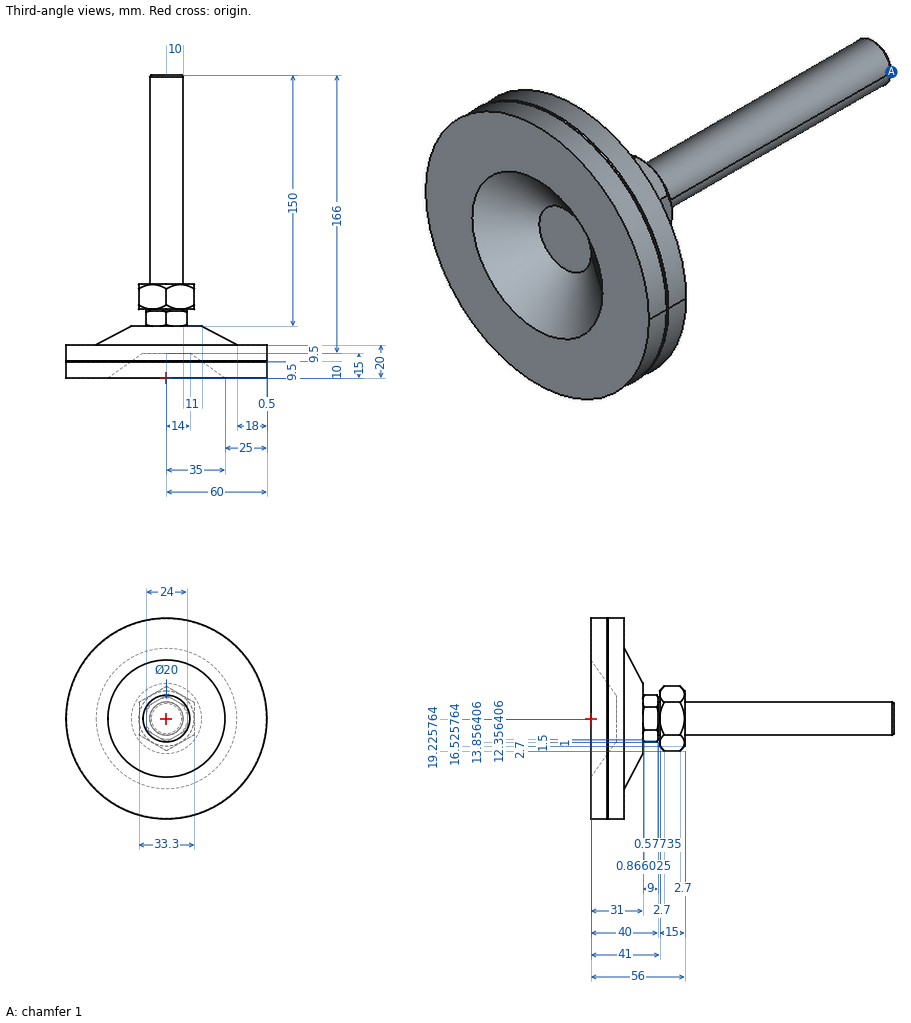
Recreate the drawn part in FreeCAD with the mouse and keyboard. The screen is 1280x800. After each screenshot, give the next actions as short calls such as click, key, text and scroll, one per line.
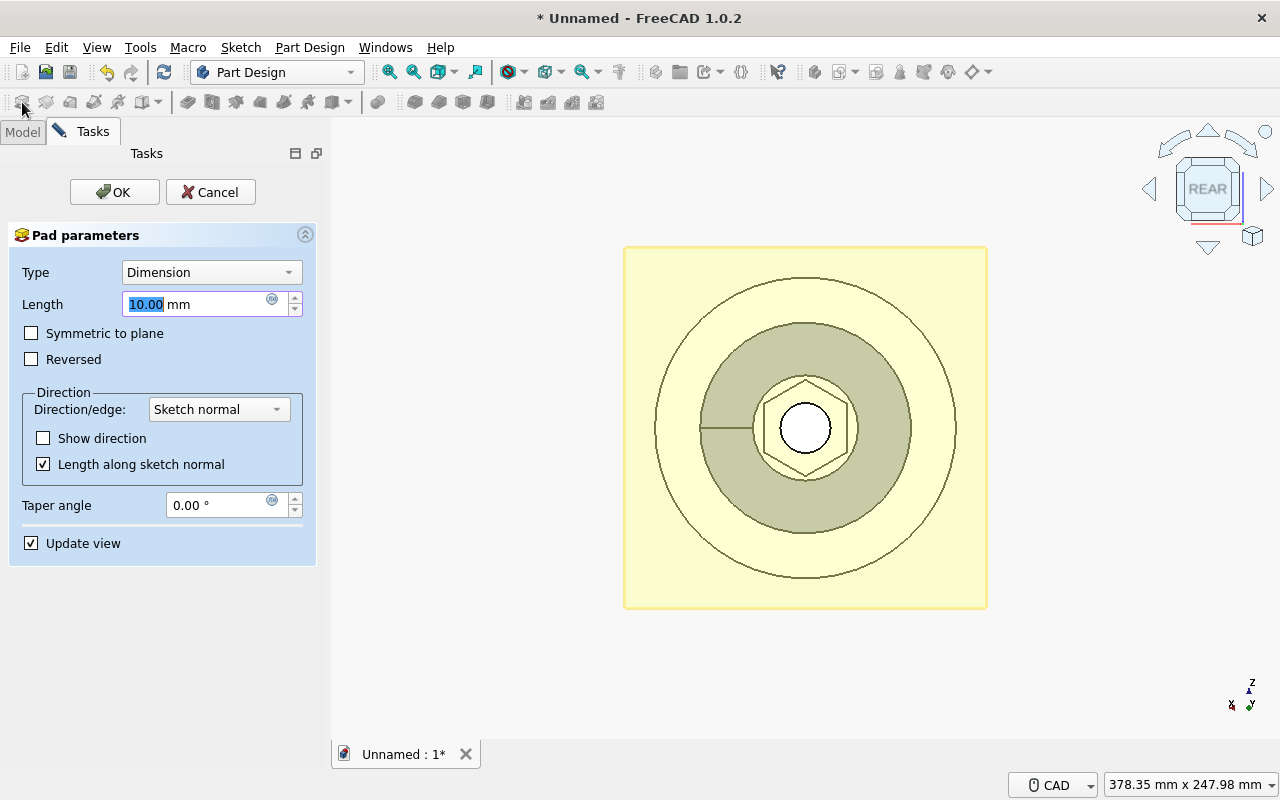
text(15)
key(Tab)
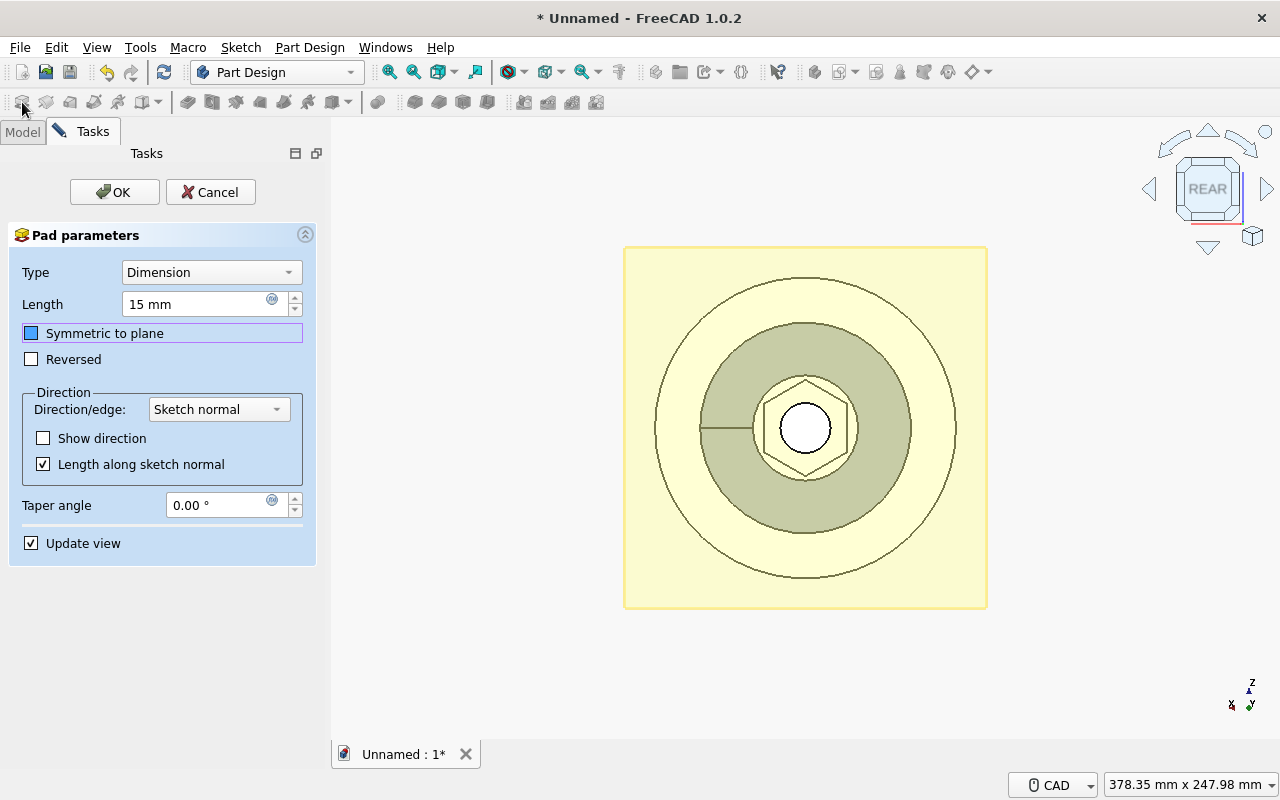
click(115, 192)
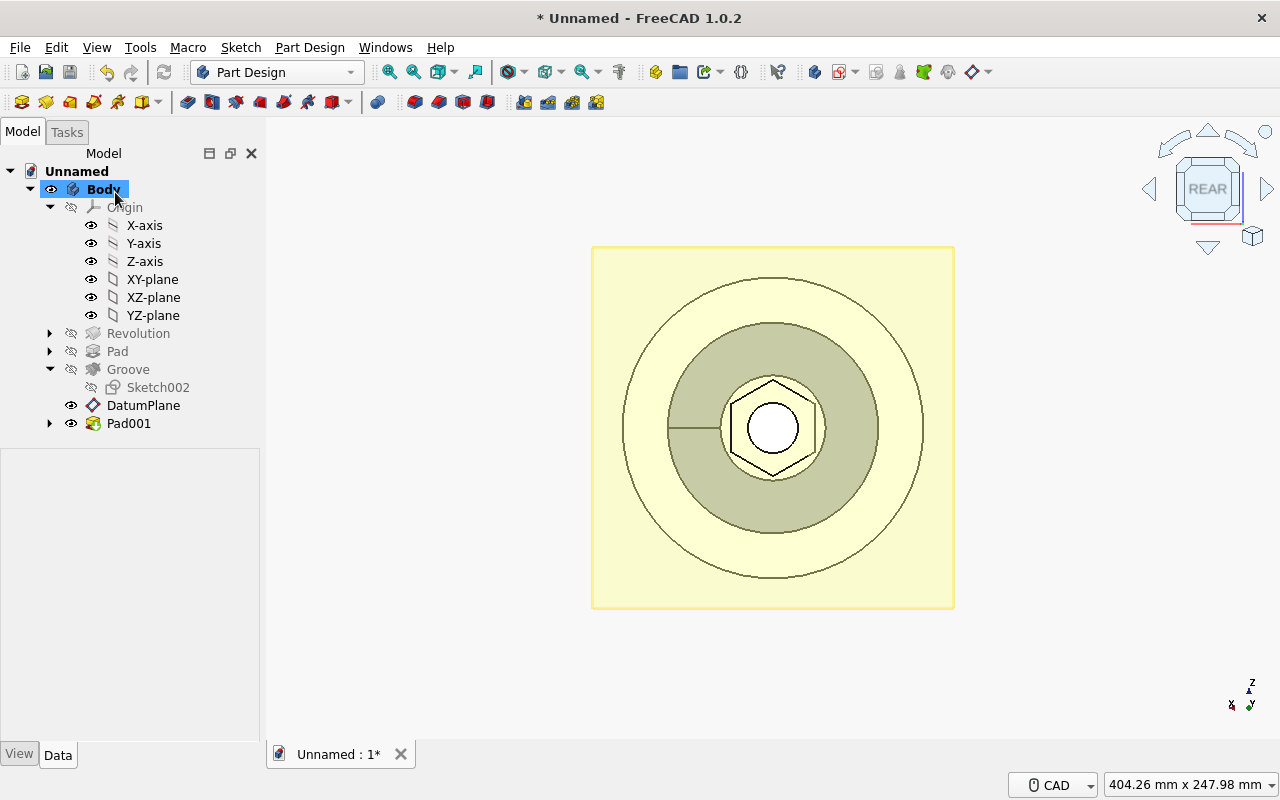
click(116, 405)
key(space)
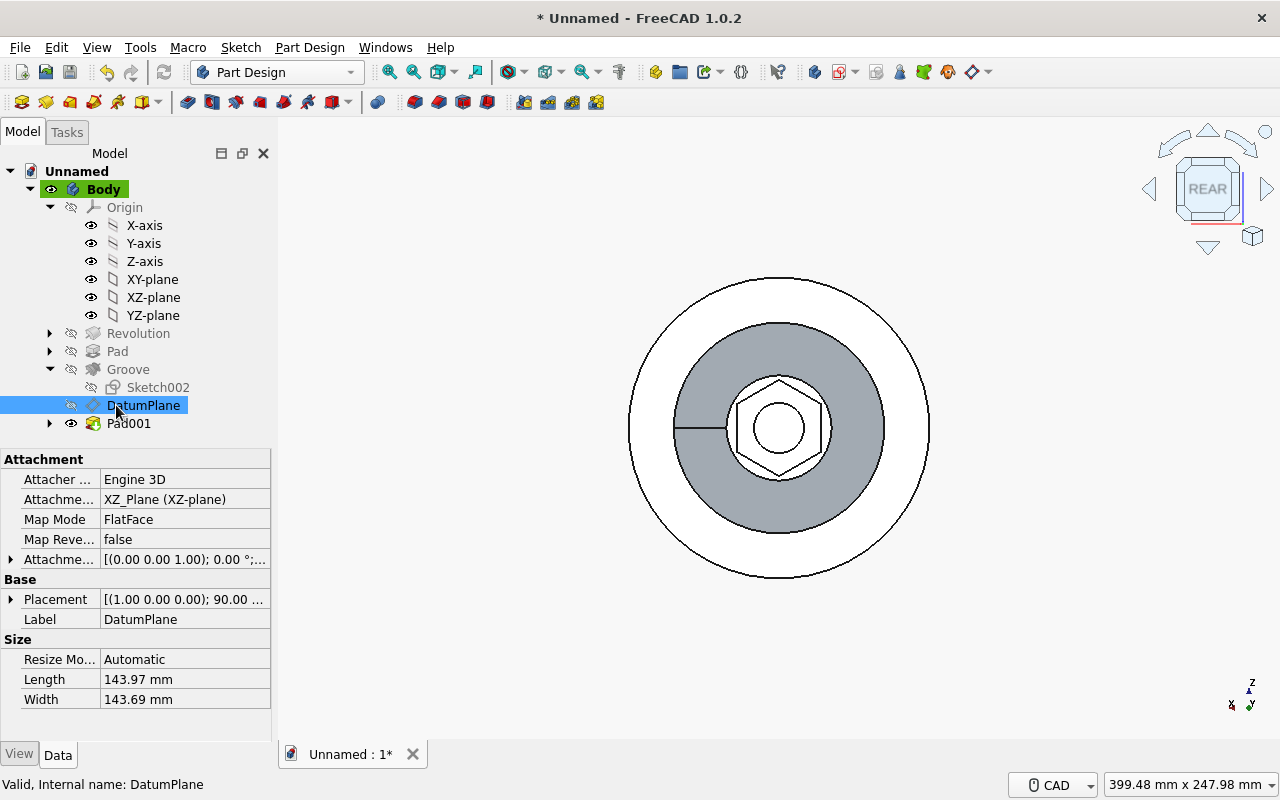
click(318, 699)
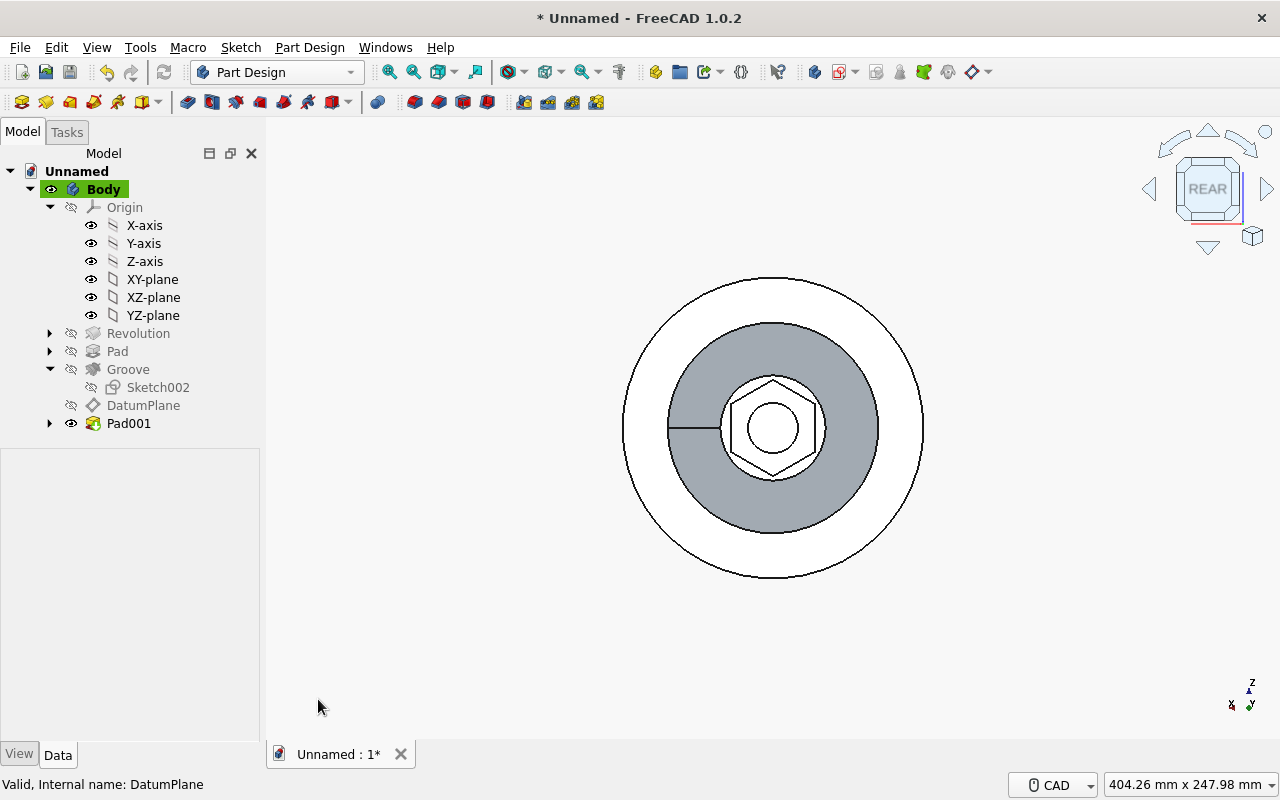
click(840, 72)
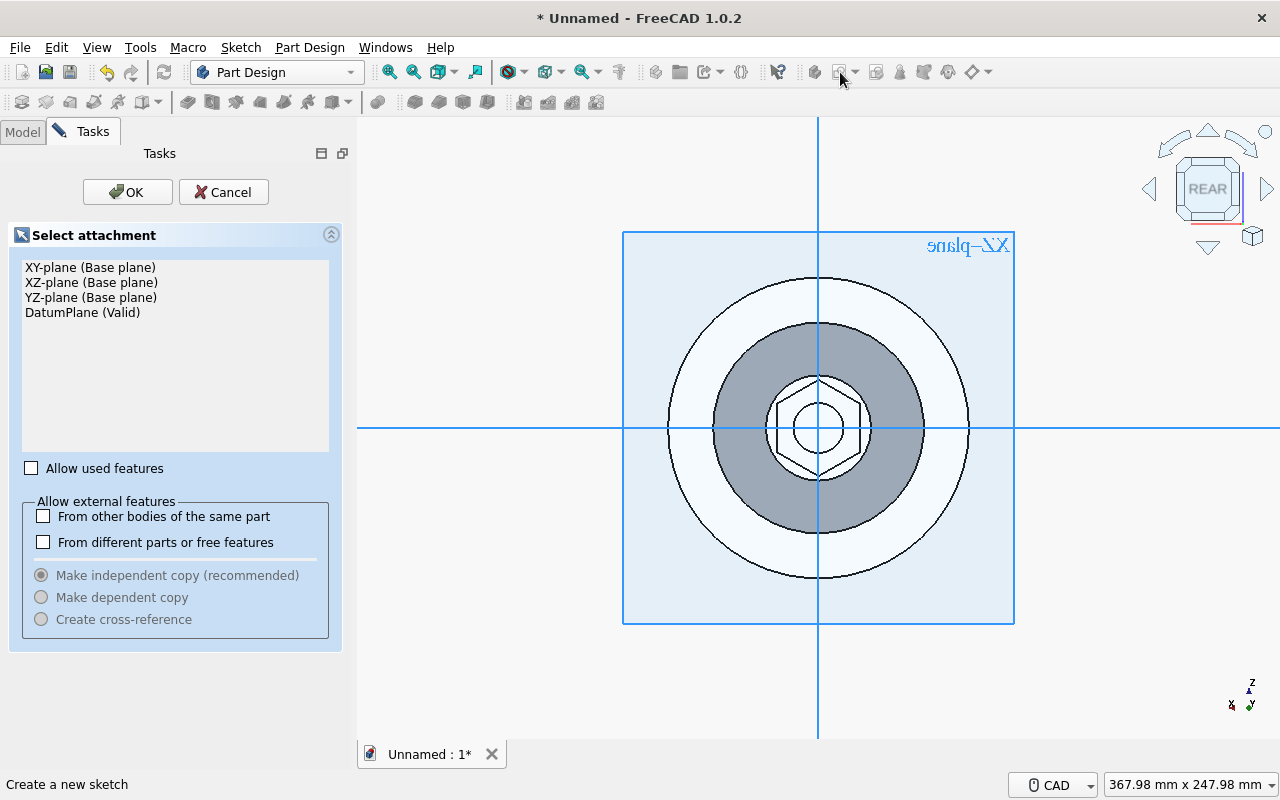
click(82, 298)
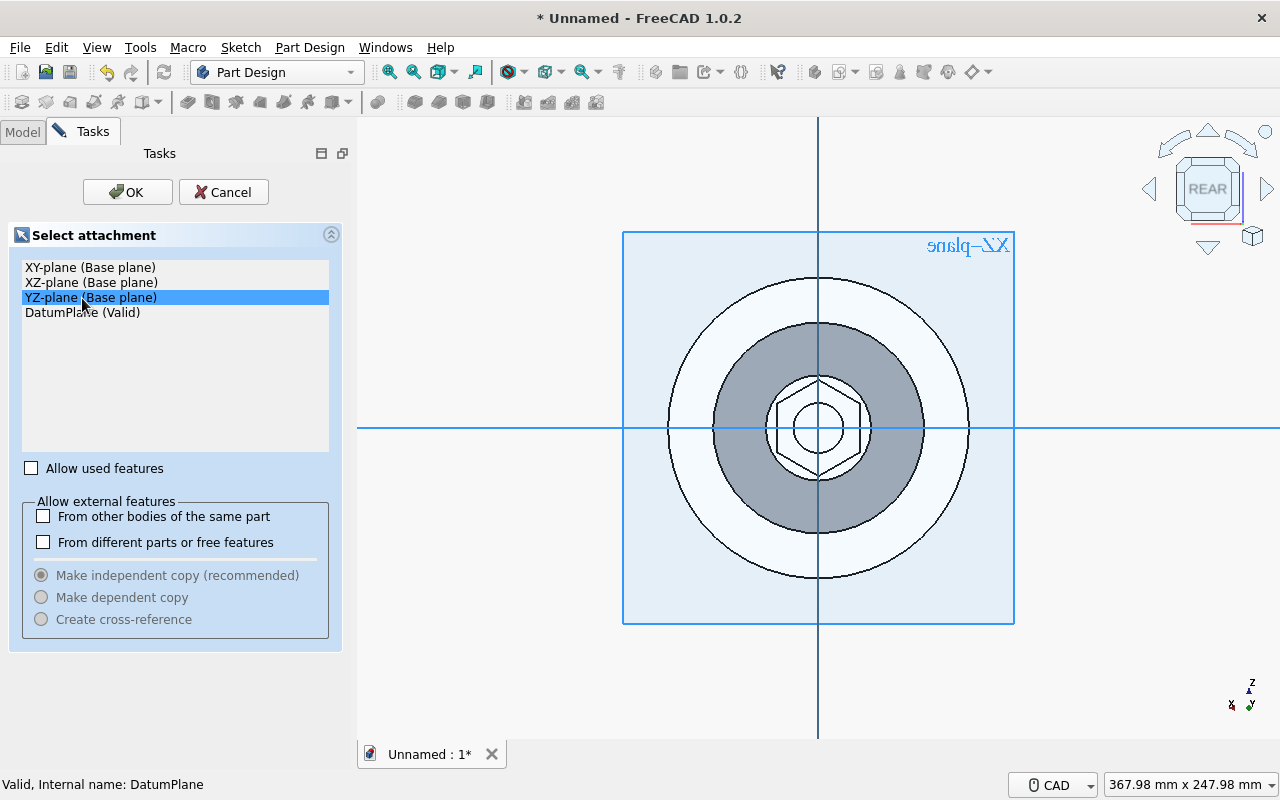
click(128, 192)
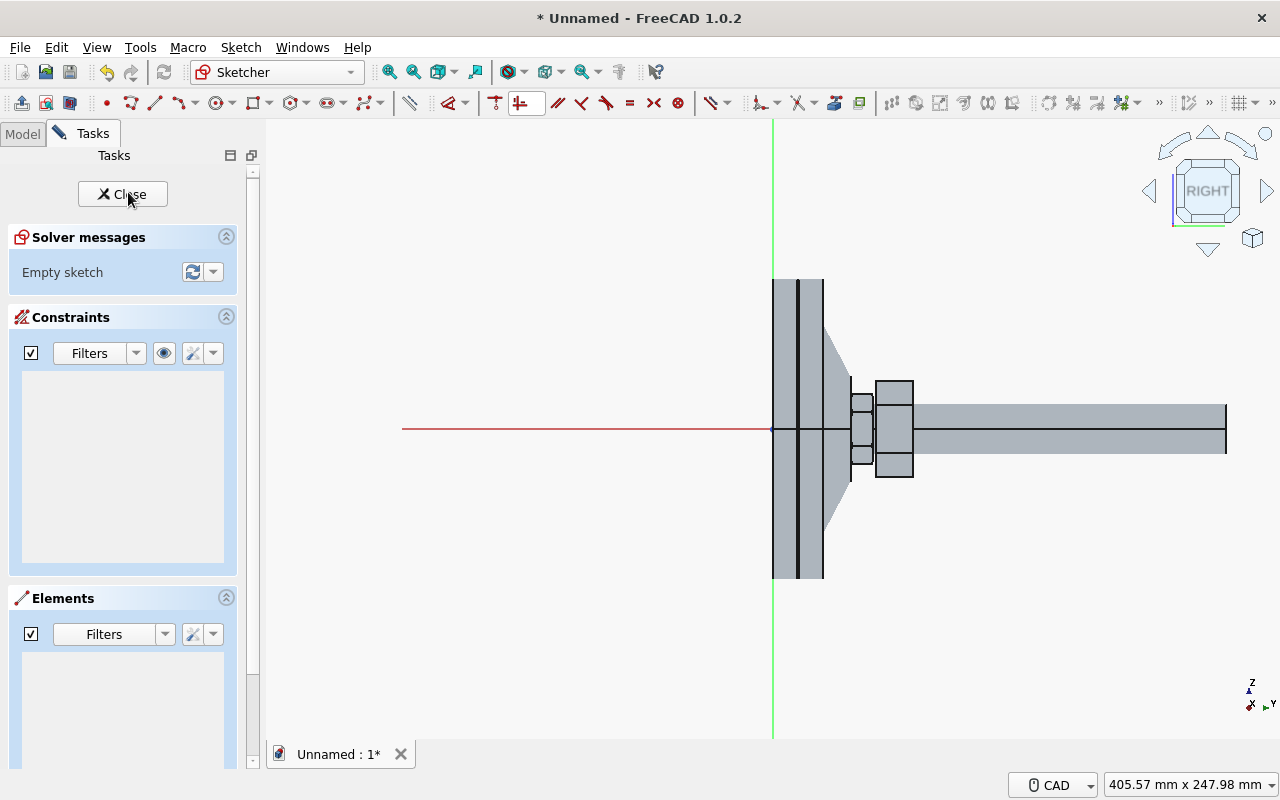
click(70, 104)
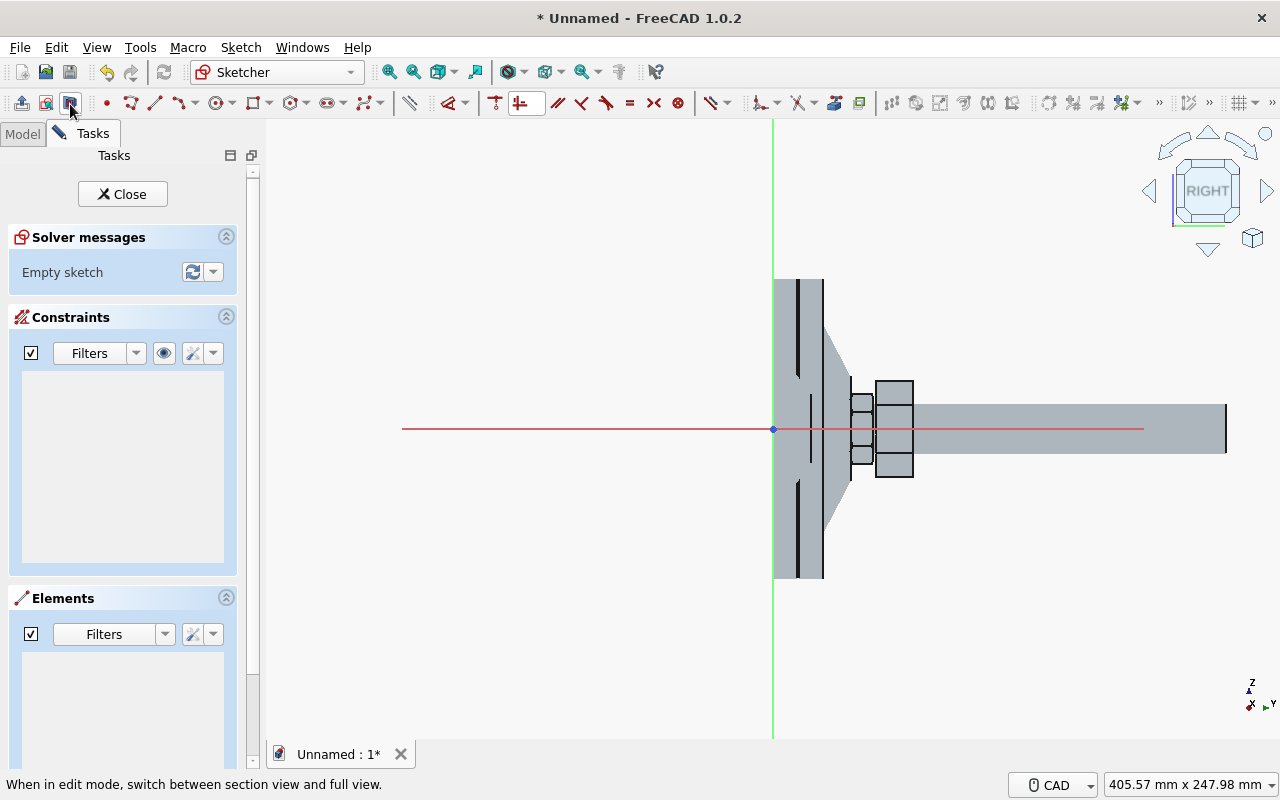
scroll(907, 477, up, 14)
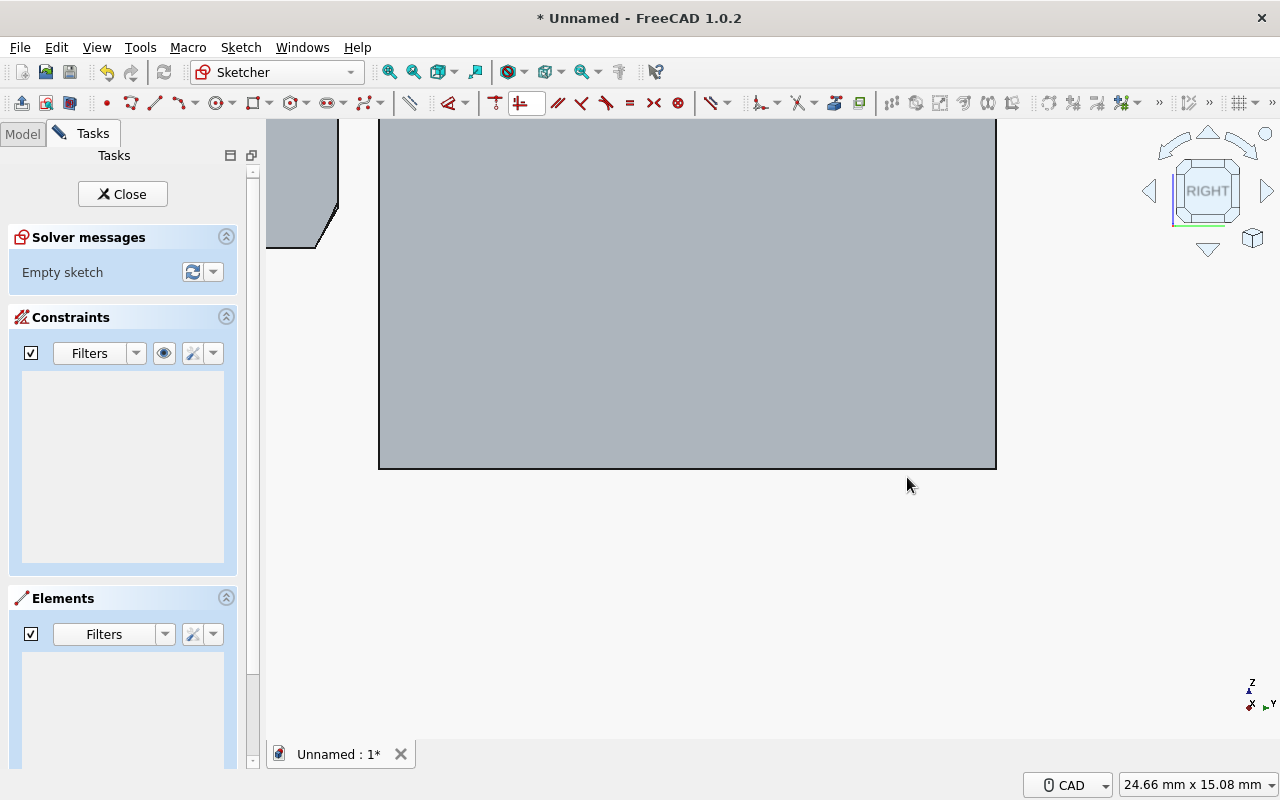
click(132, 104)